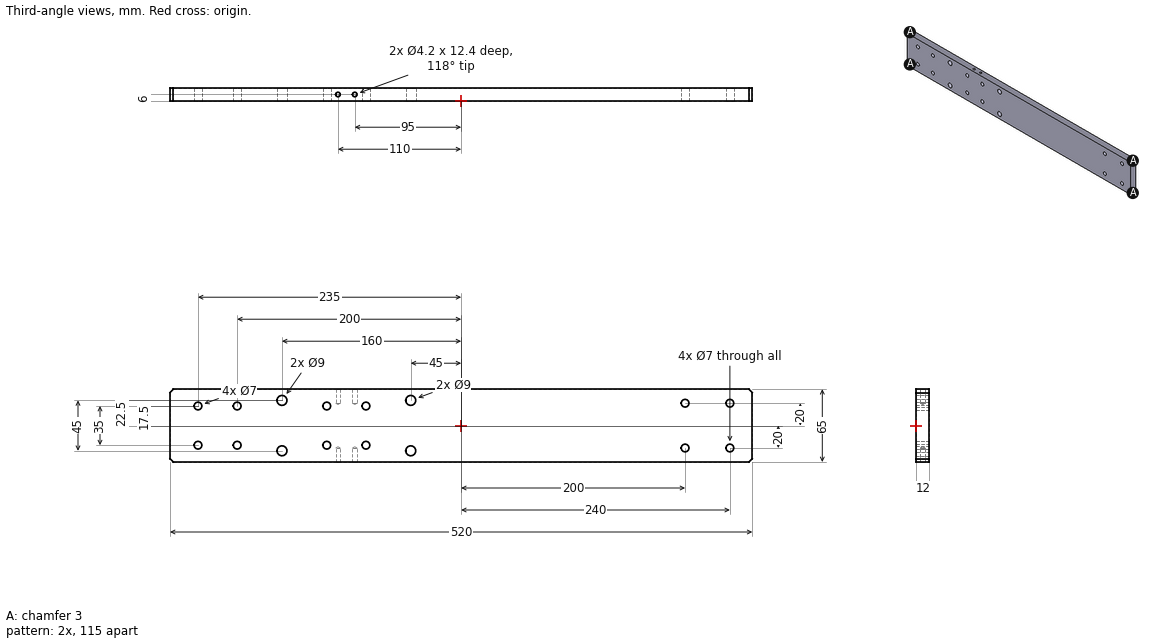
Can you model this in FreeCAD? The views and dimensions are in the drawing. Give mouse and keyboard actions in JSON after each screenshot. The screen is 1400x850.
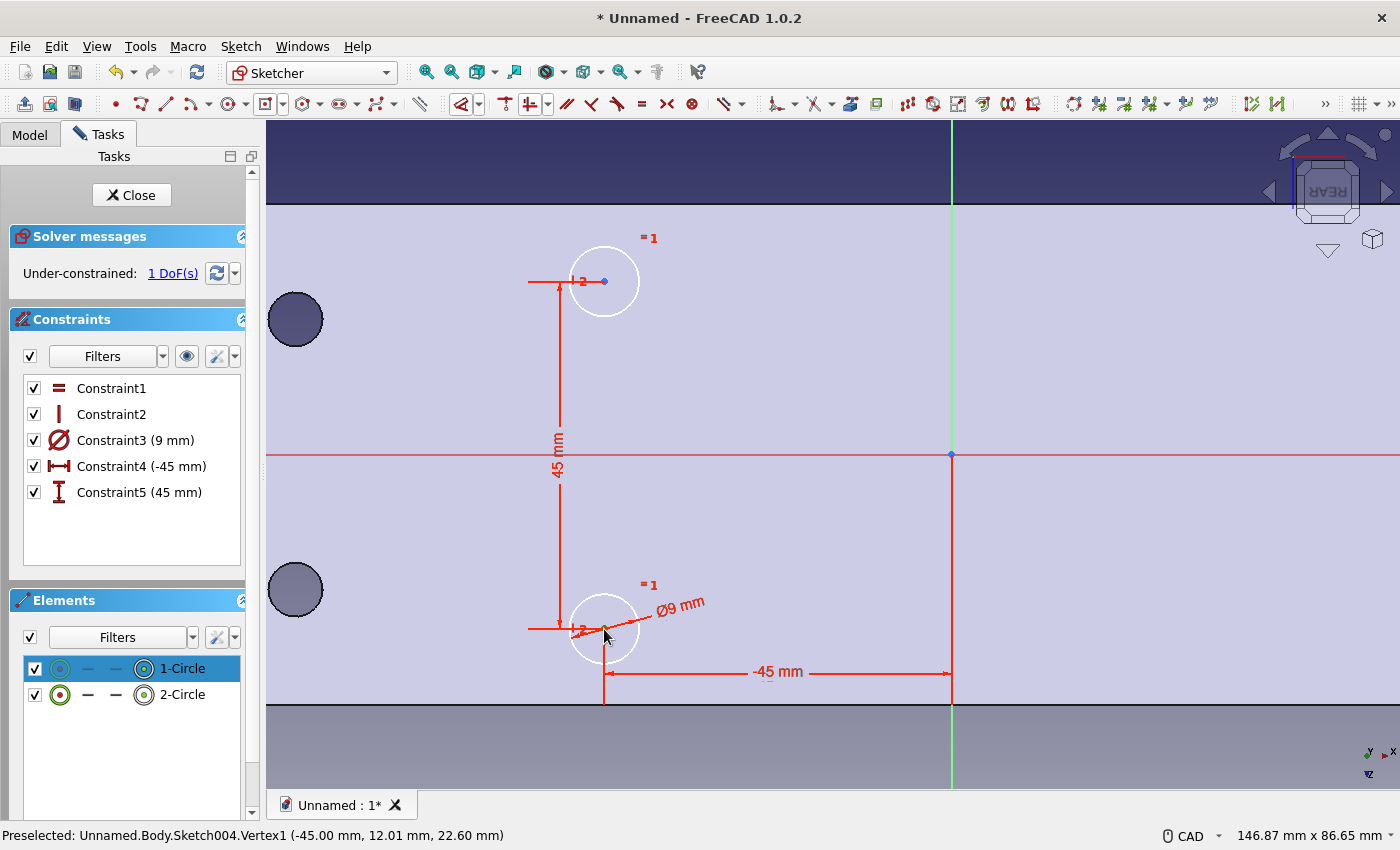
{"action": "left_click", "coordinate": [478, 104]}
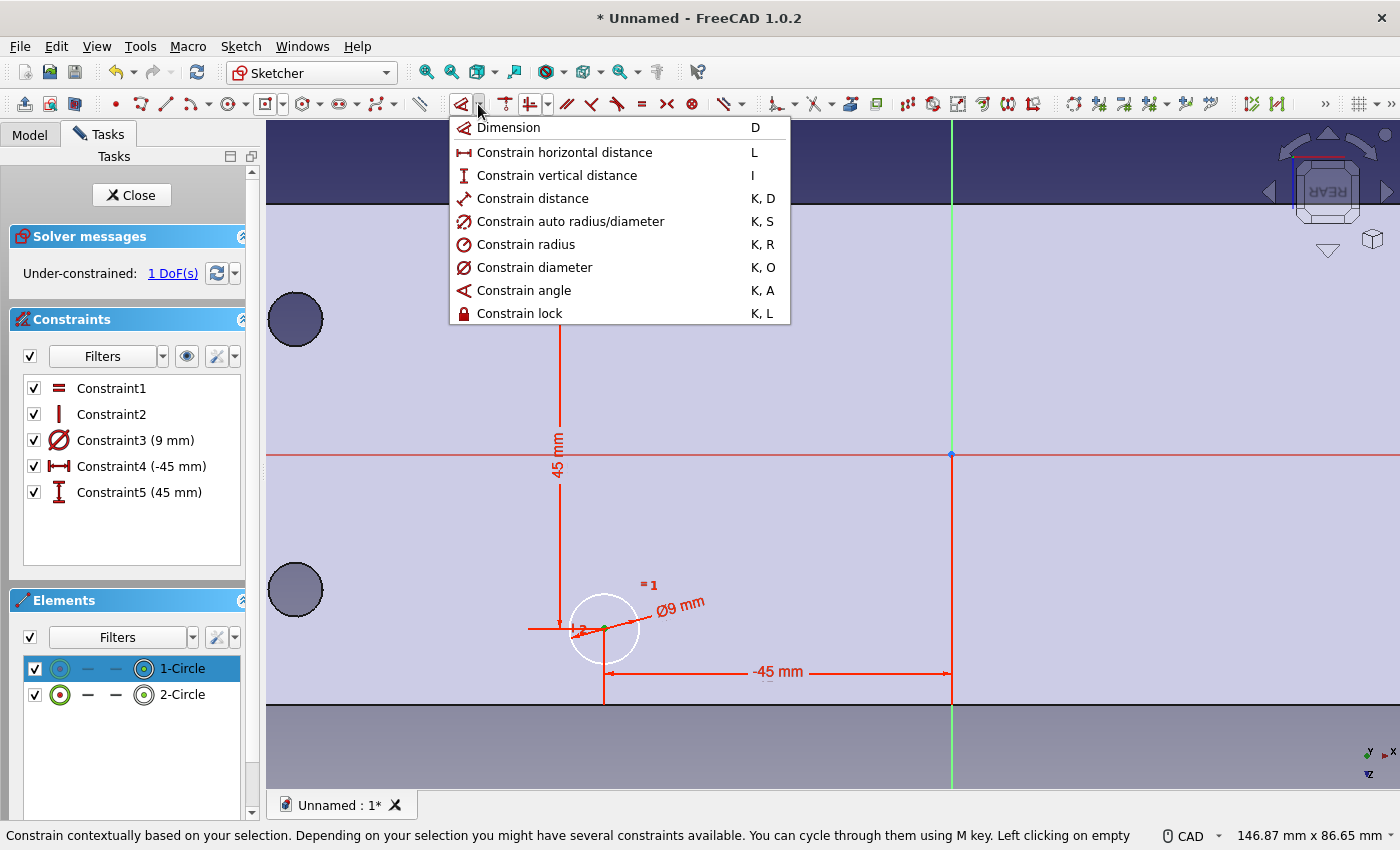
{"action": "left_click", "coordinate": [620, 176]}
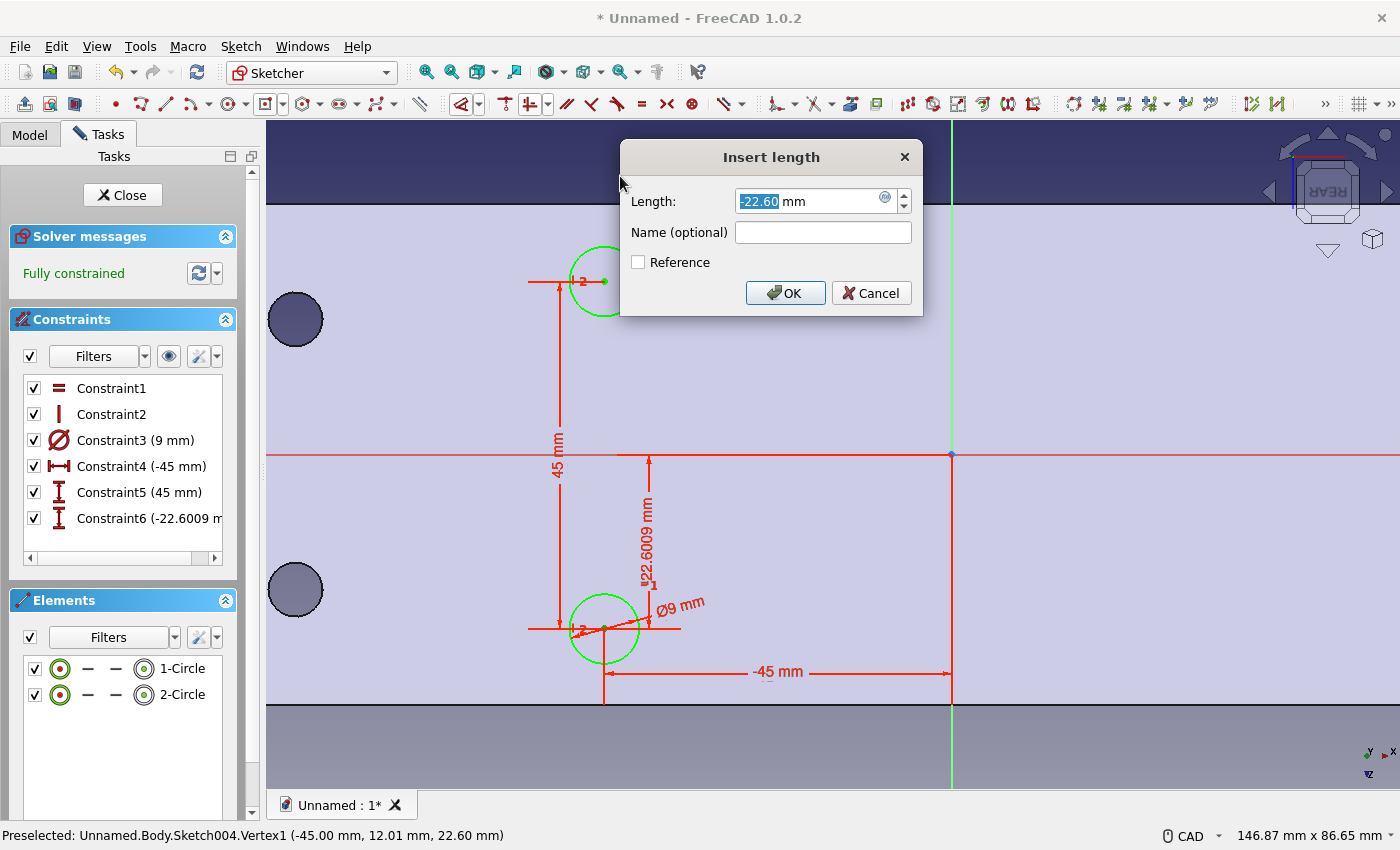
{"action": "type", "text": "-22.5"}
{"action": "key", "text": "Return"}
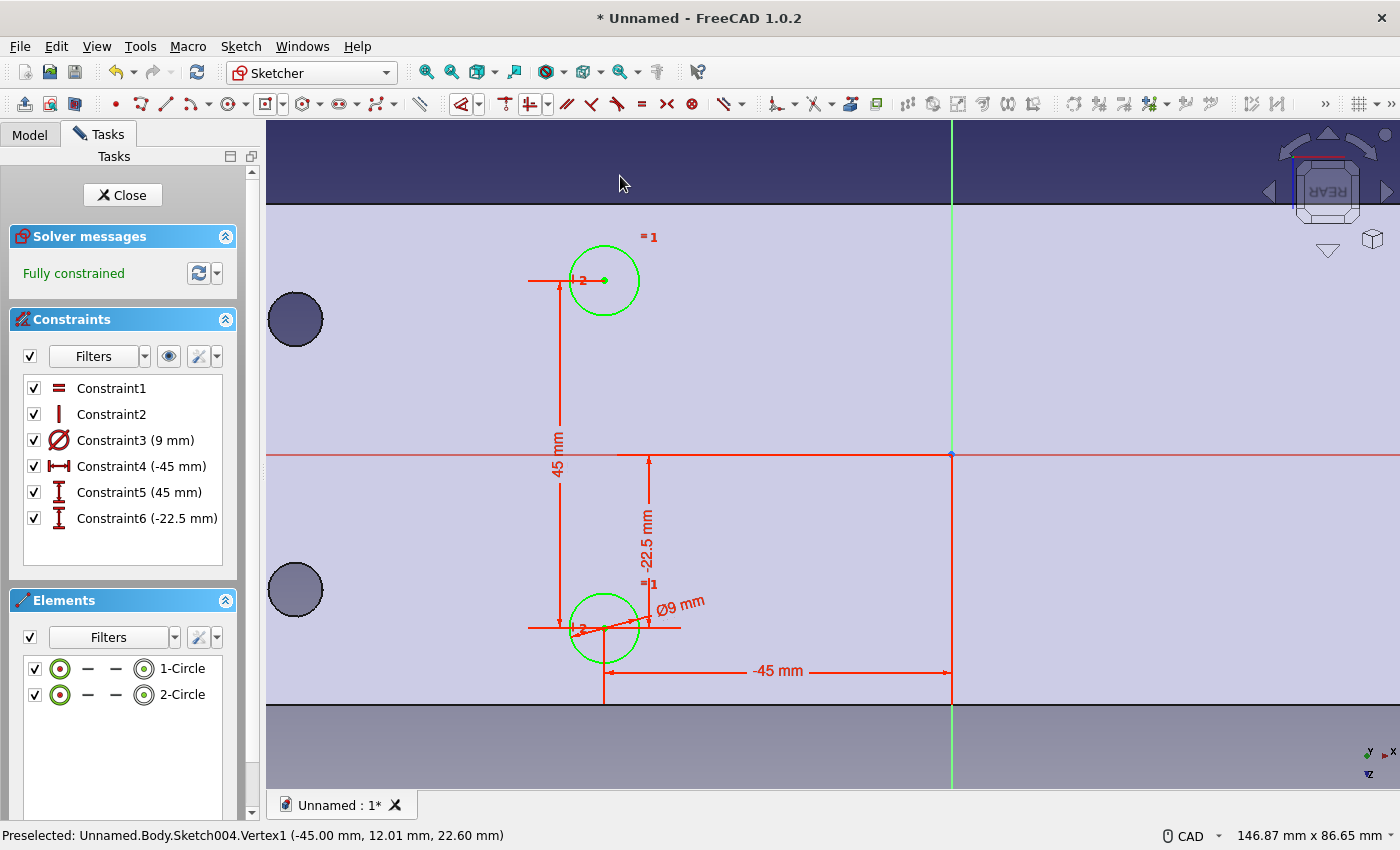
{"action": "left_click", "coordinate": [123, 195]}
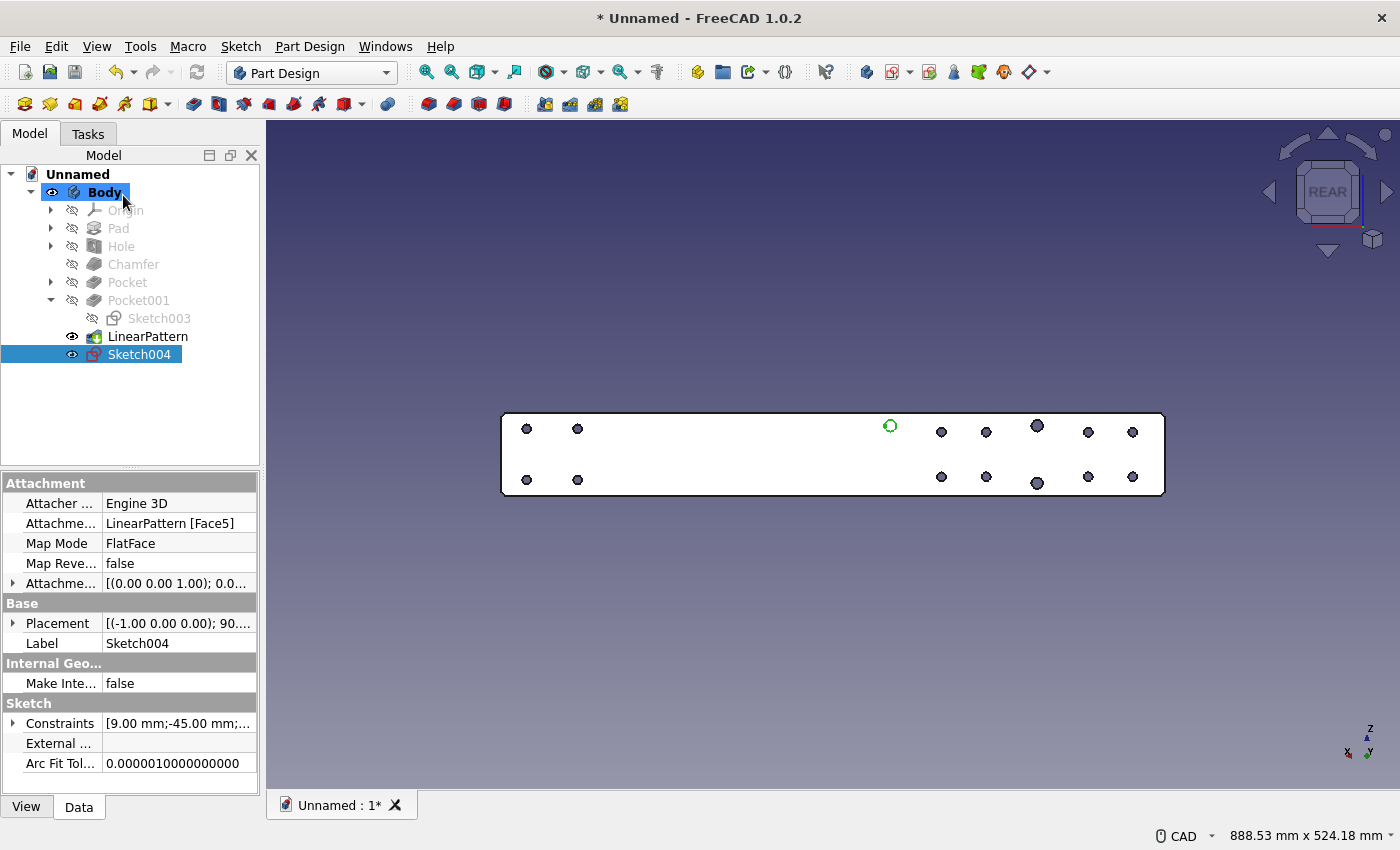
{"action": "left_click", "coordinate": [194, 104]}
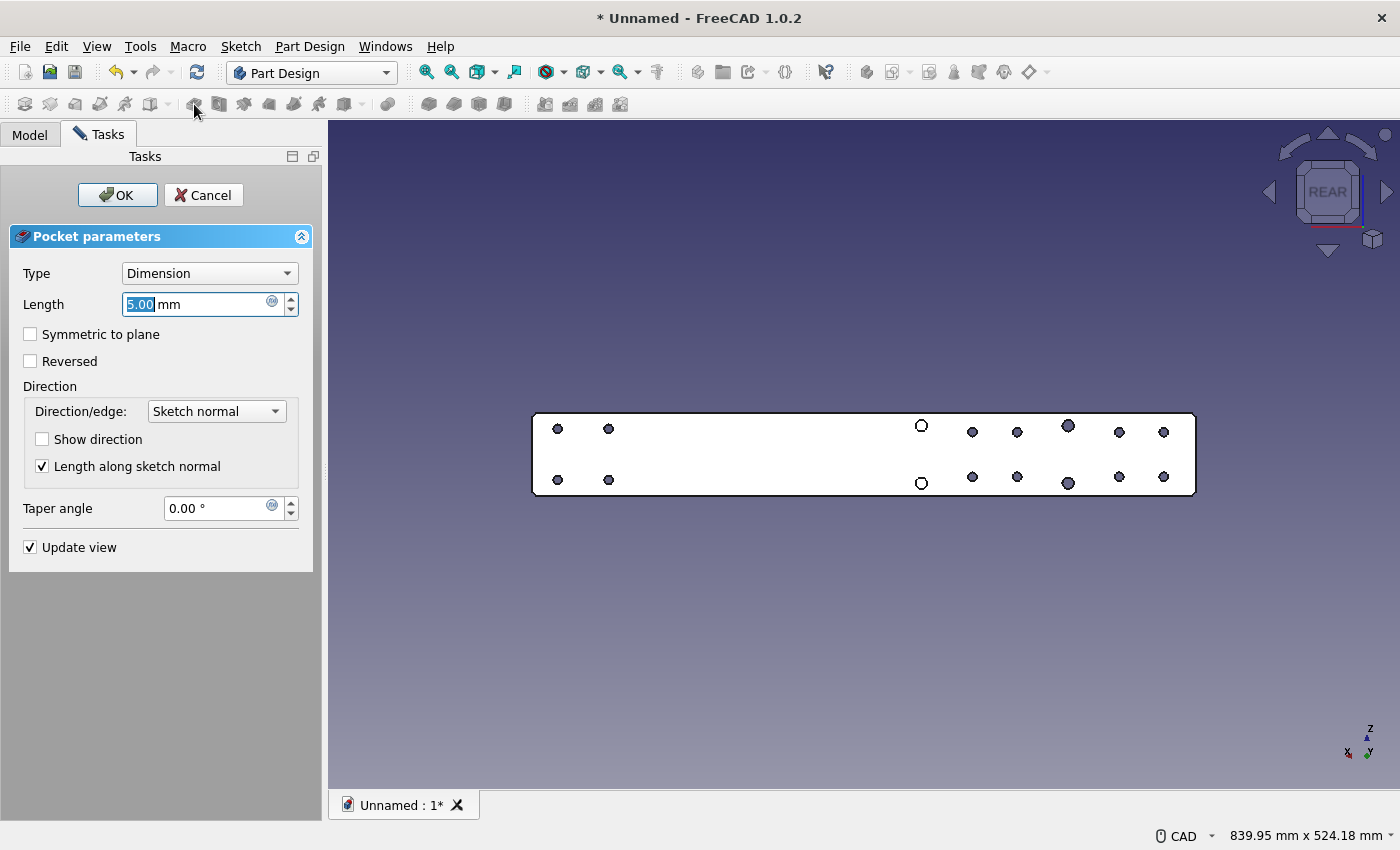
{"action": "left_click", "coordinate": [210, 274]}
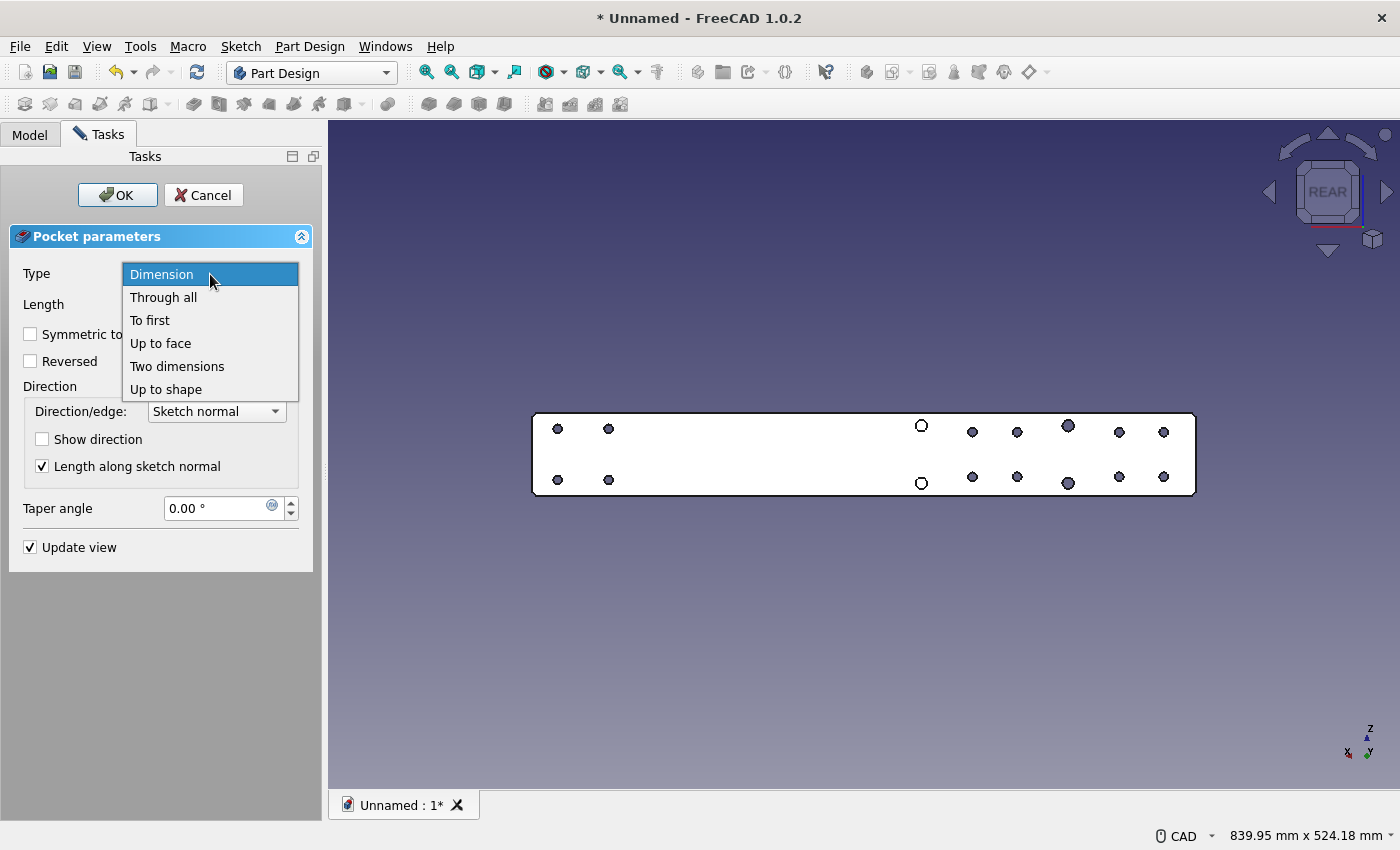
{"action": "left_click", "coordinate": [208, 298]}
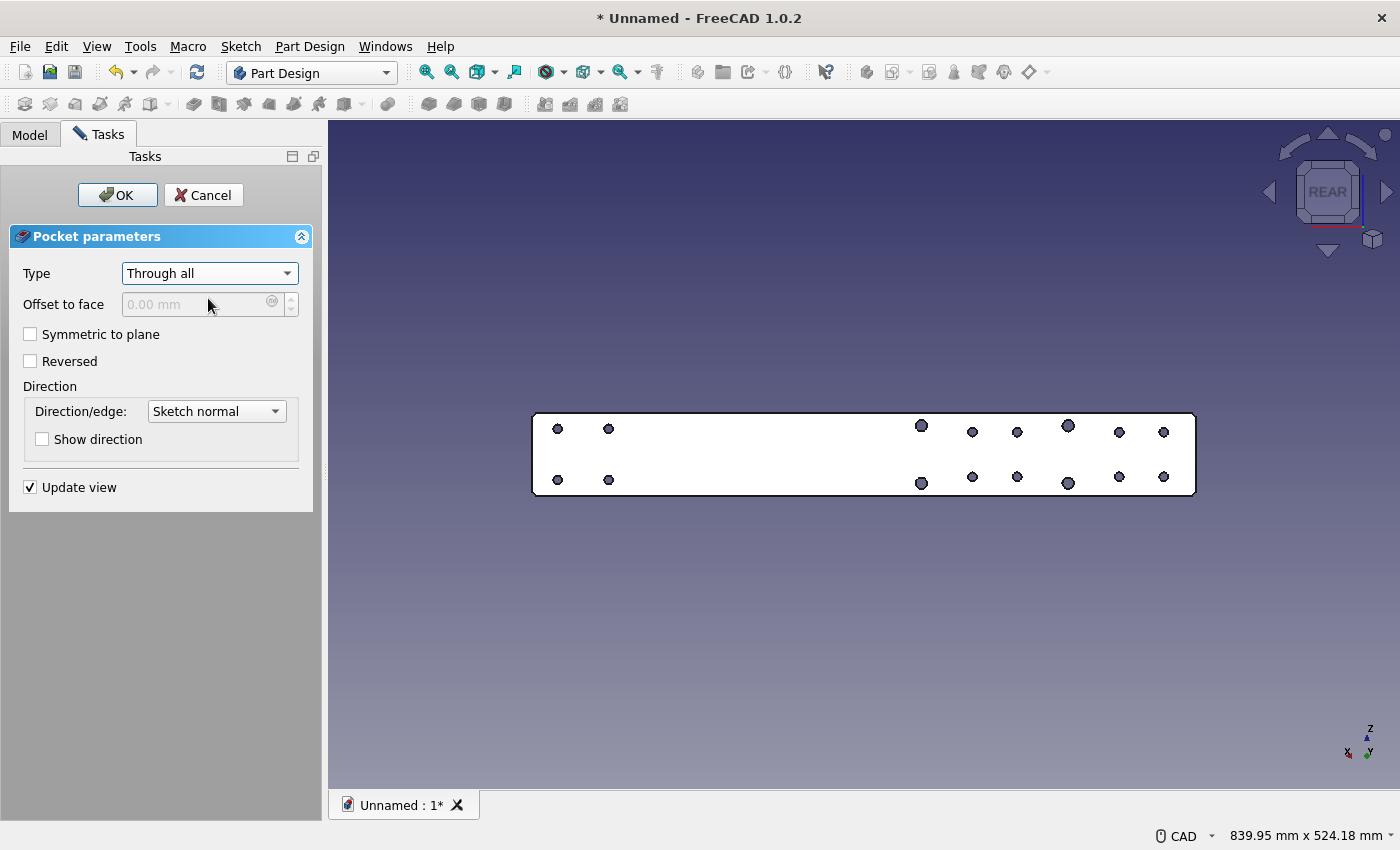
{"action": "left_click", "coordinate": [118, 195]}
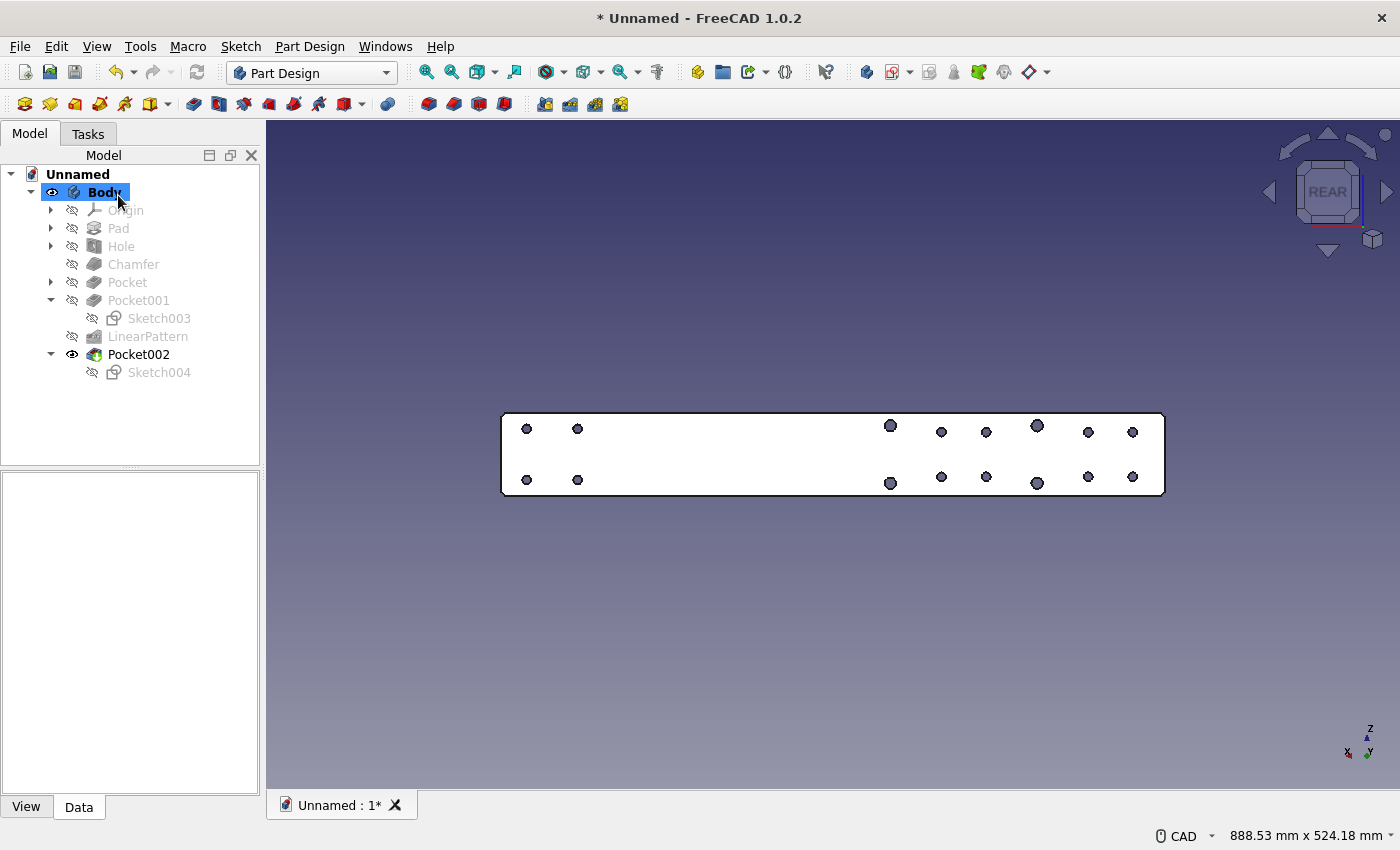
{"action": "key", "text": "5"}